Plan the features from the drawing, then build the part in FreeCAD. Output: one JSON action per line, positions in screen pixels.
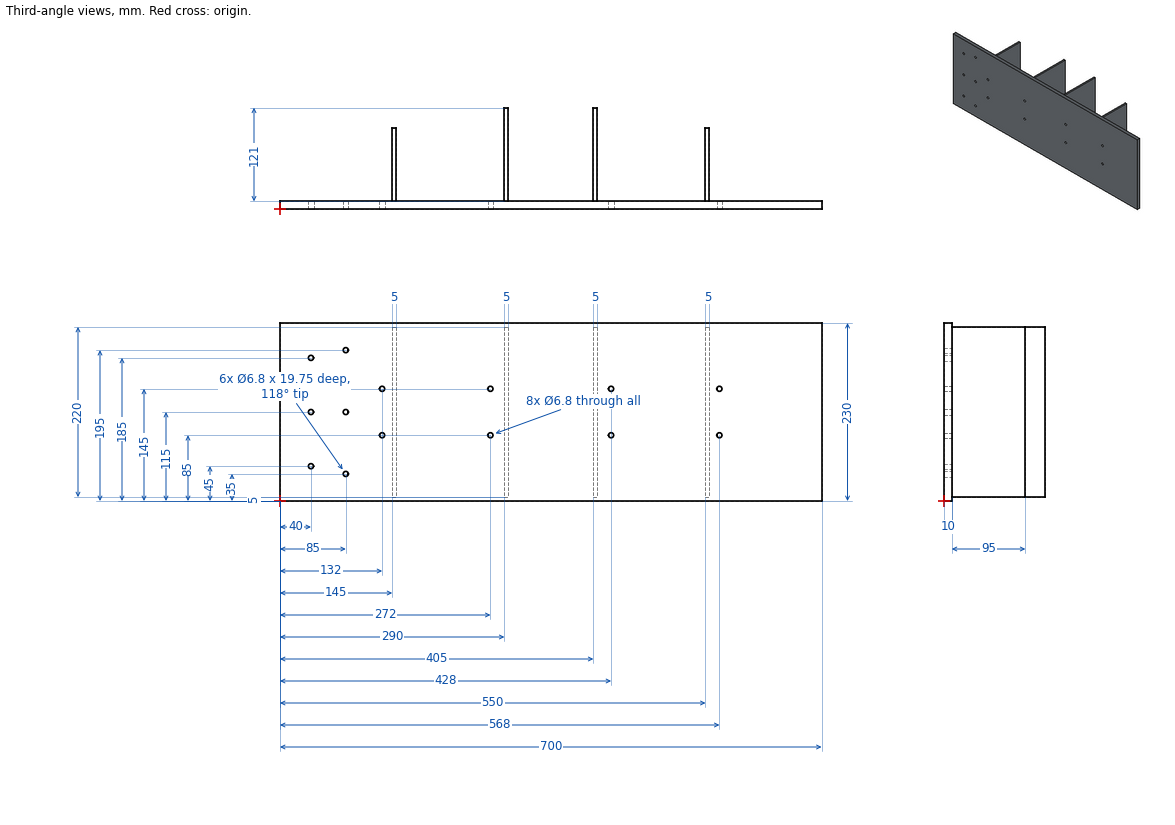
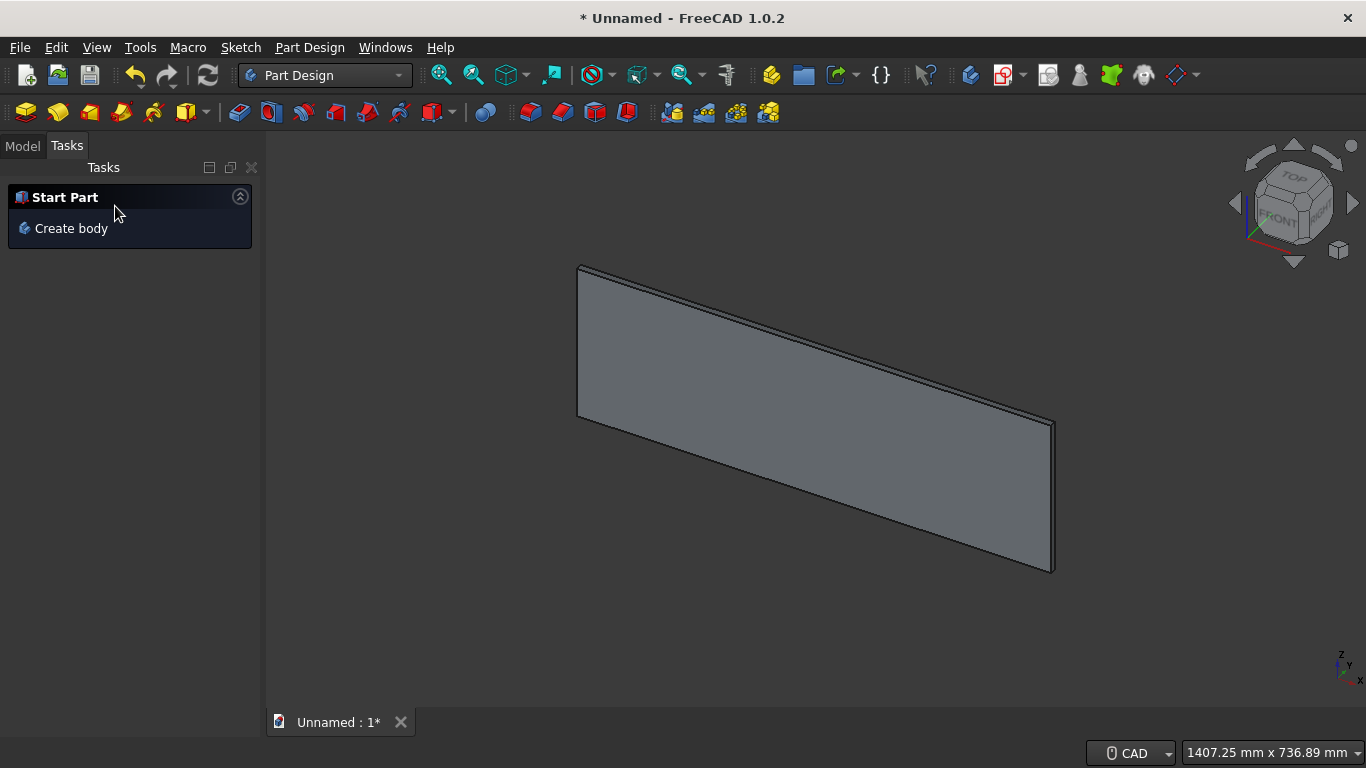
{"action": "key", "text": "4"}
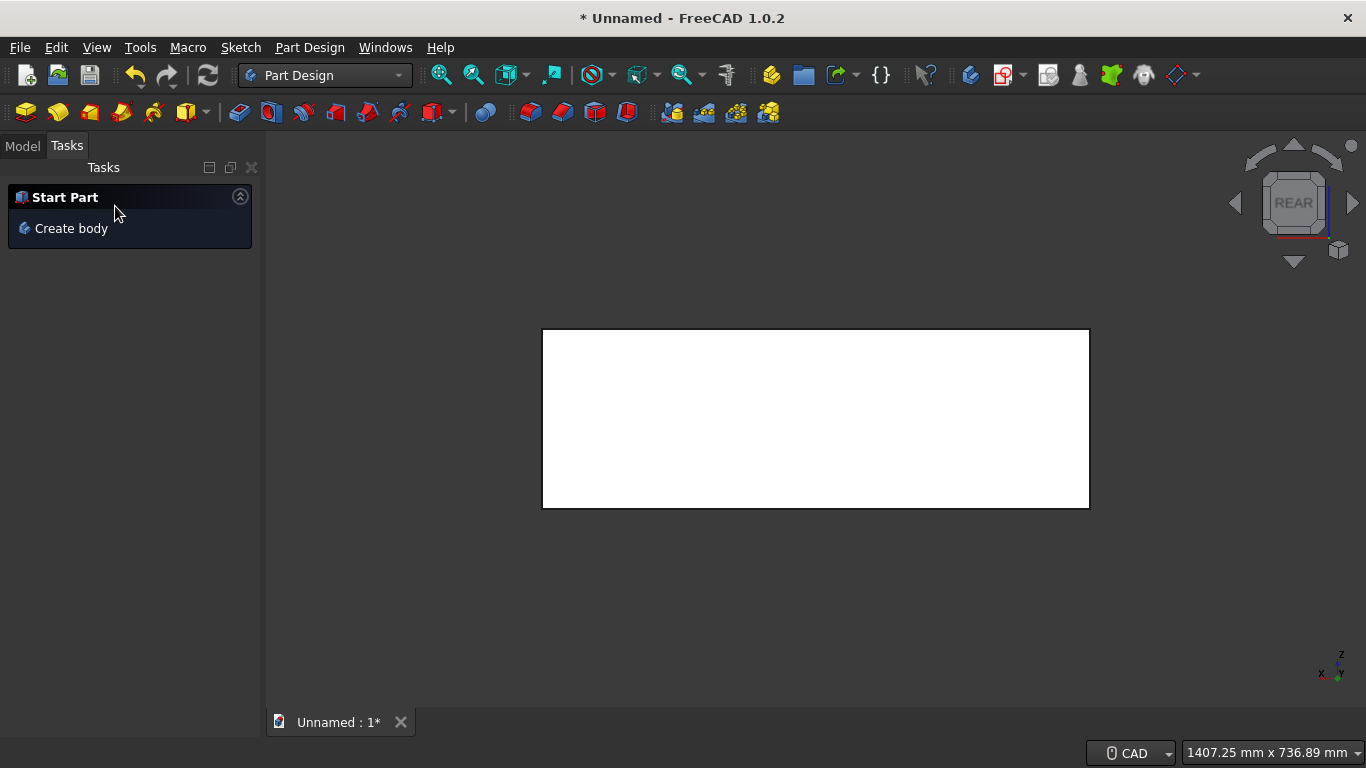
{"action": "left_click", "coordinate": [660, 418]}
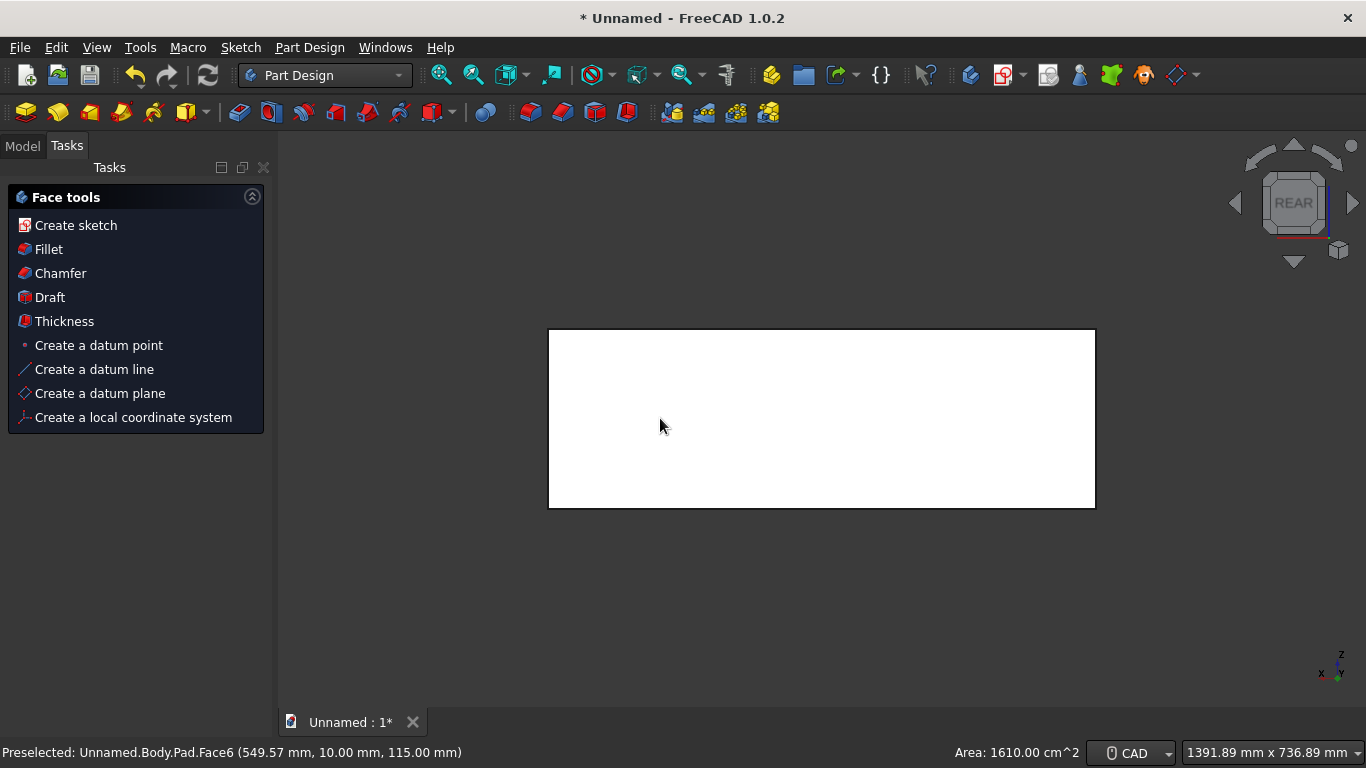
{"action": "left_click", "coordinate": [1004, 76]}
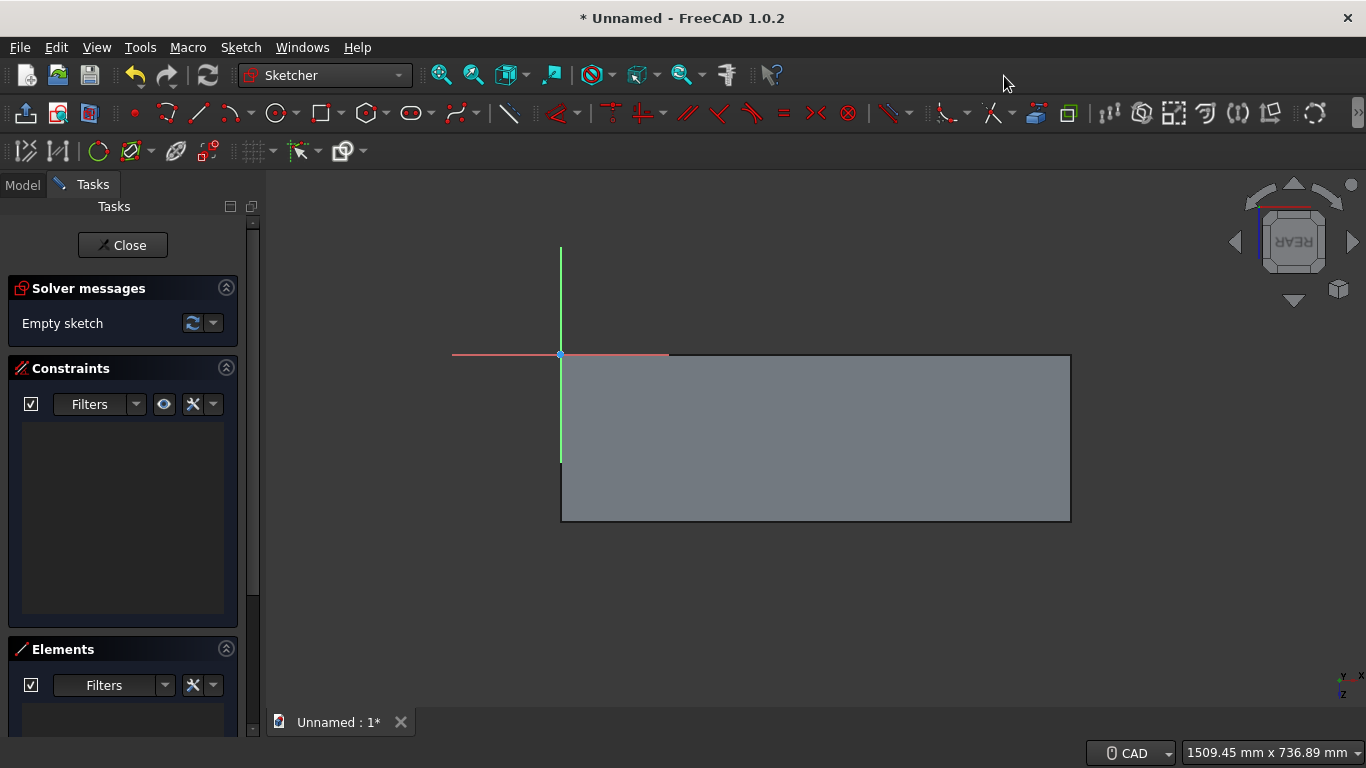
{"action": "scroll", "coordinate": [813, 348], "scroll_direction": "up", "scroll_amount": 2}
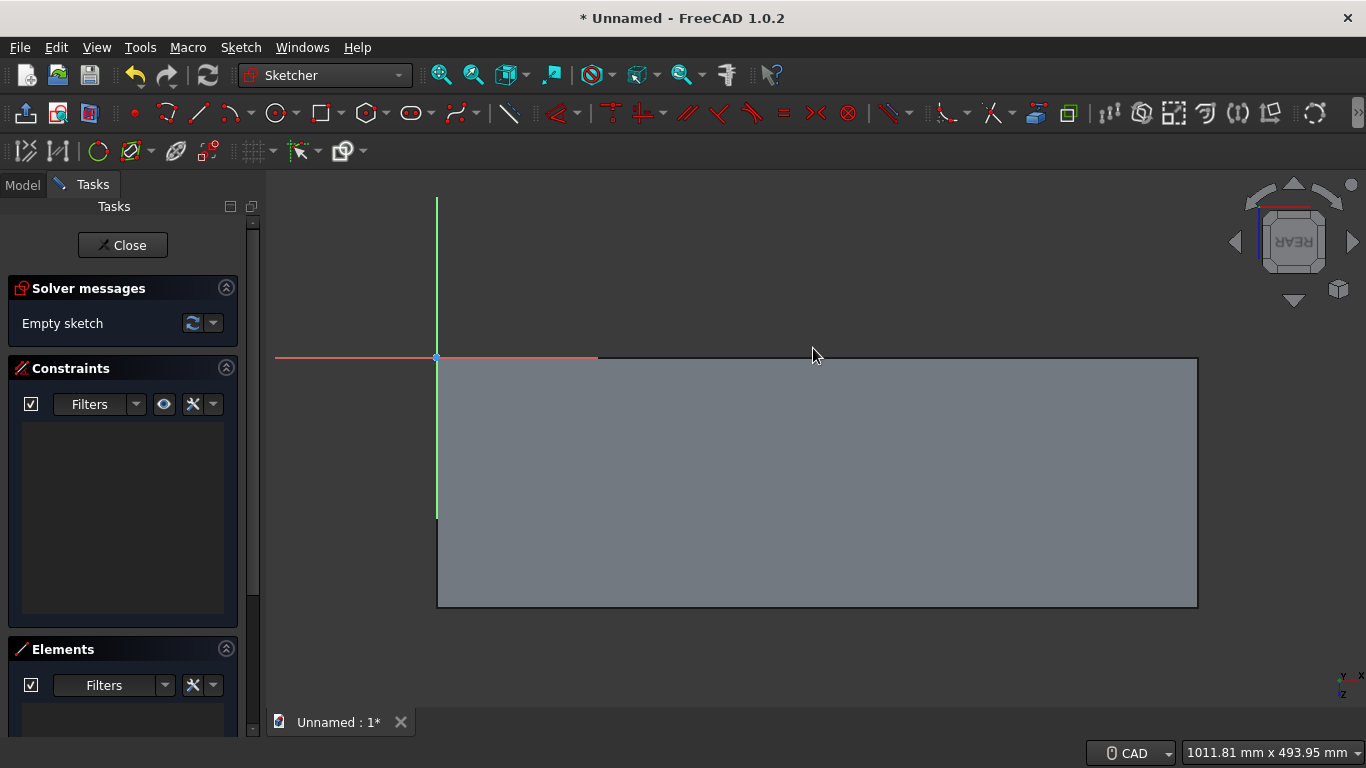
{"action": "key", "text": "g c"}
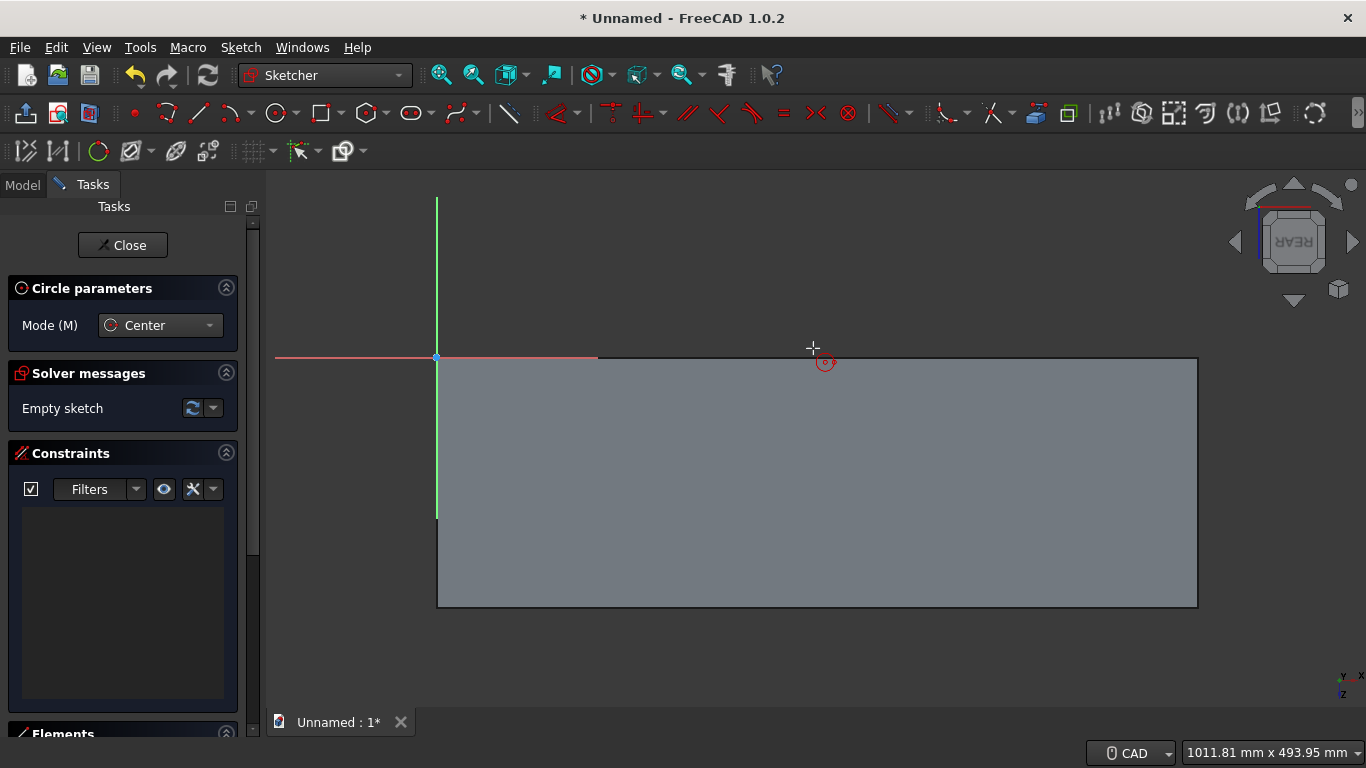
{"action": "scroll", "coordinate": [732, 450], "scroll_direction": "up", "scroll_amount": 10}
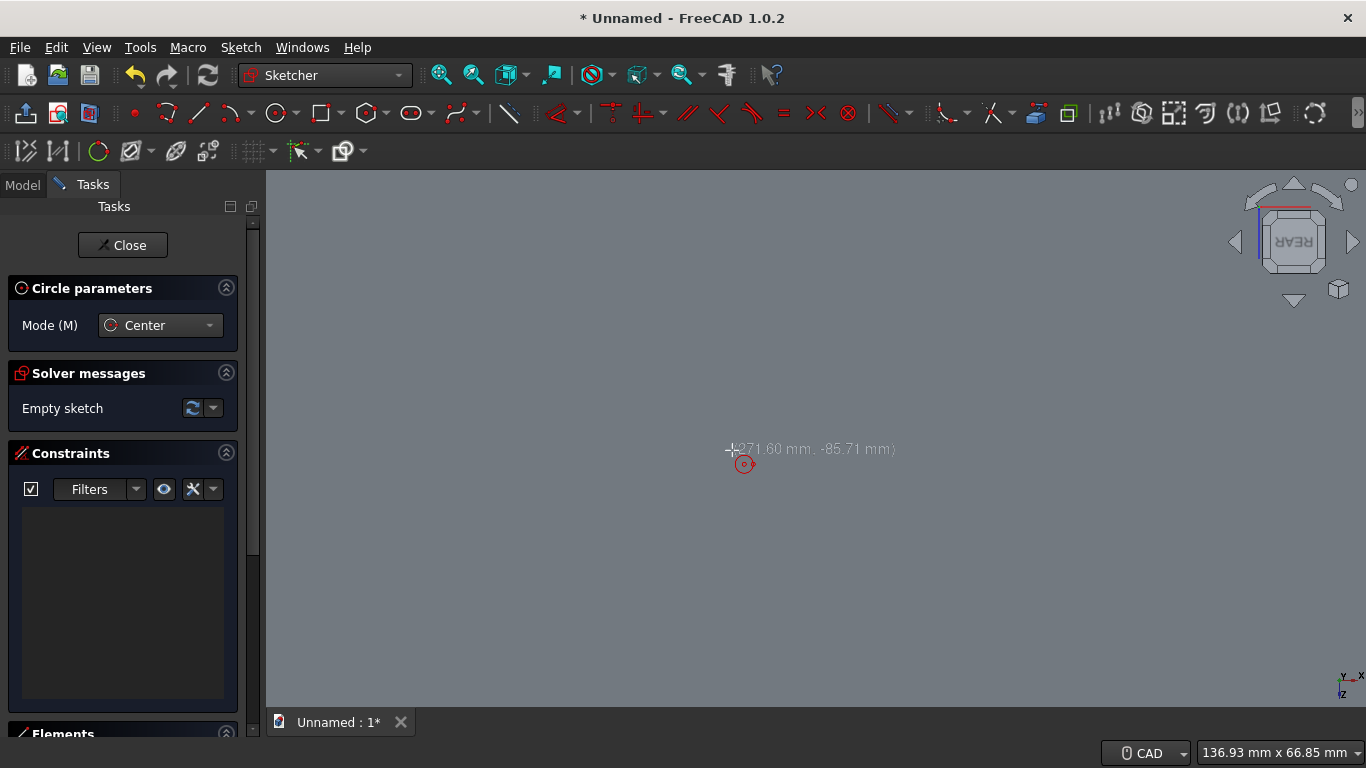
{"action": "scroll", "coordinate": [733, 451], "scroll_direction": "down", "scroll_amount": 10}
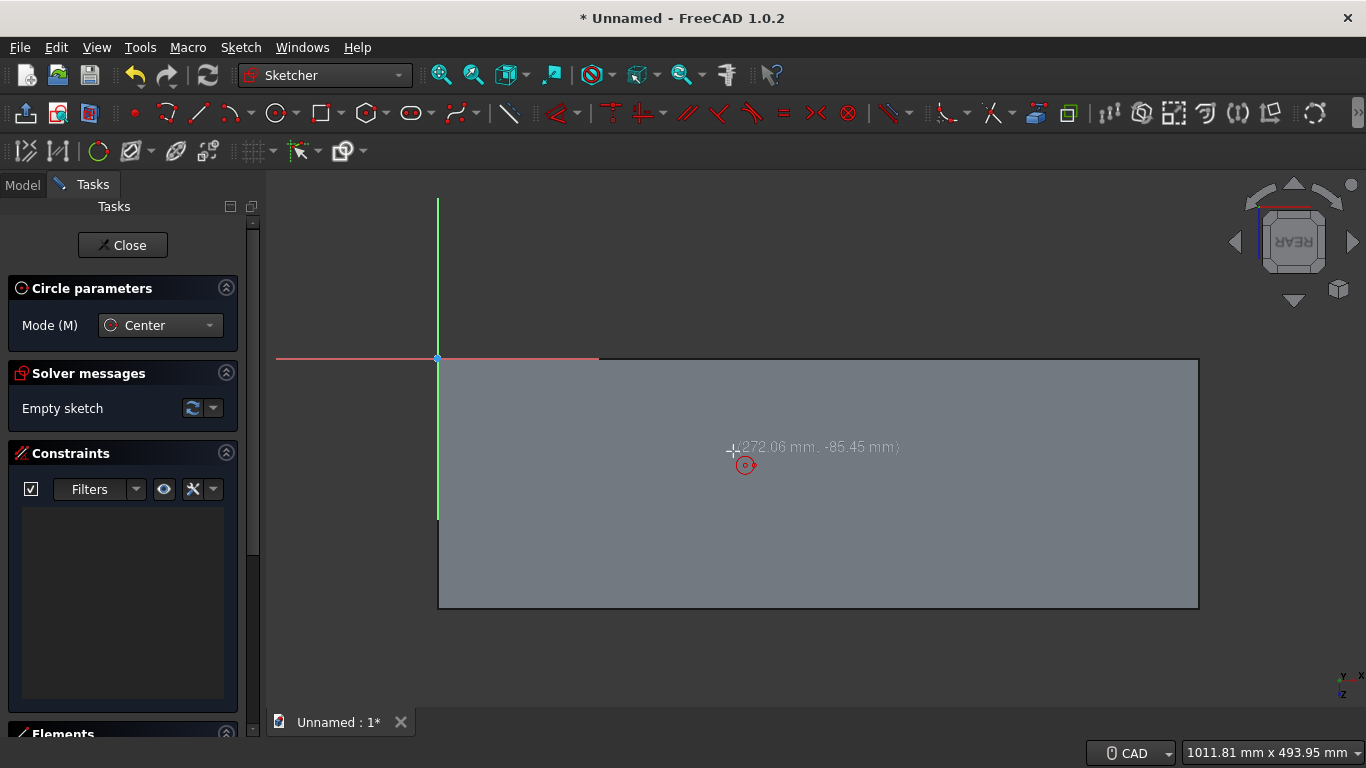
{"action": "left_click", "coordinate": [733, 451]}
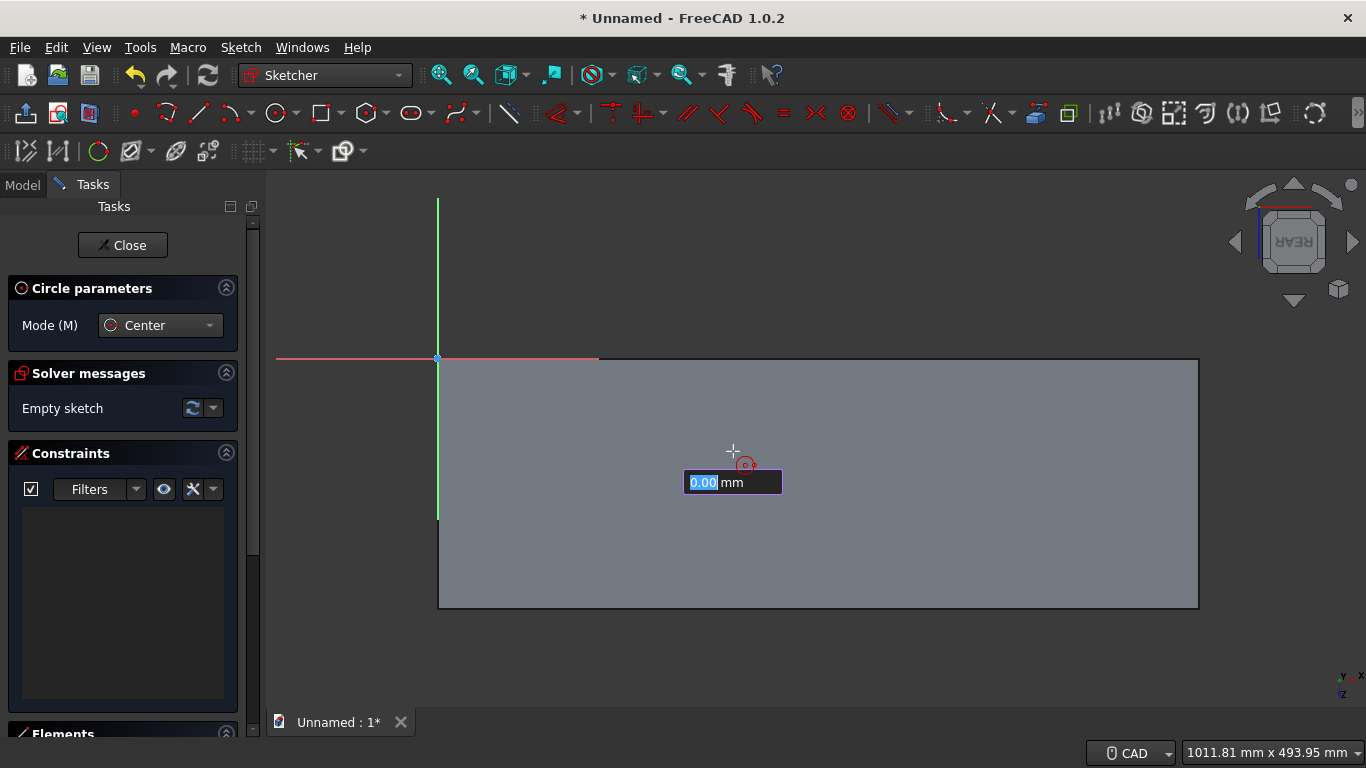
{"action": "scroll", "coordinate": [736, 448], "scroll_direction": "up", "scroll_amount": 8}